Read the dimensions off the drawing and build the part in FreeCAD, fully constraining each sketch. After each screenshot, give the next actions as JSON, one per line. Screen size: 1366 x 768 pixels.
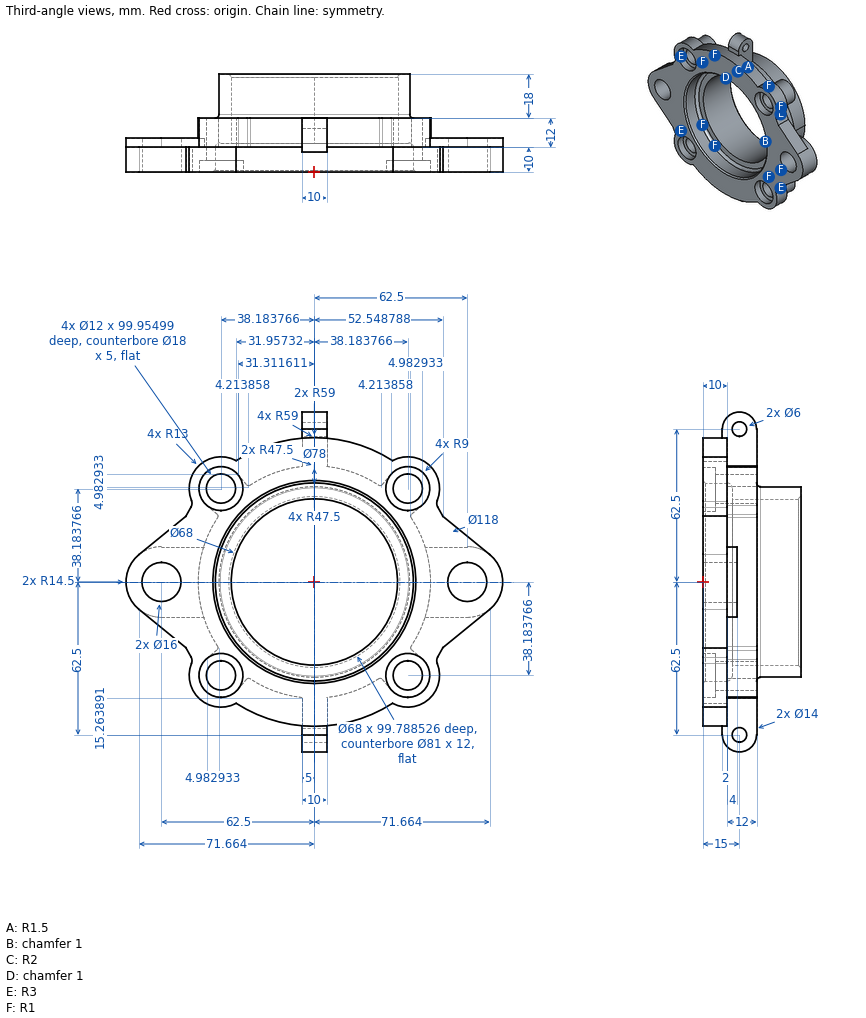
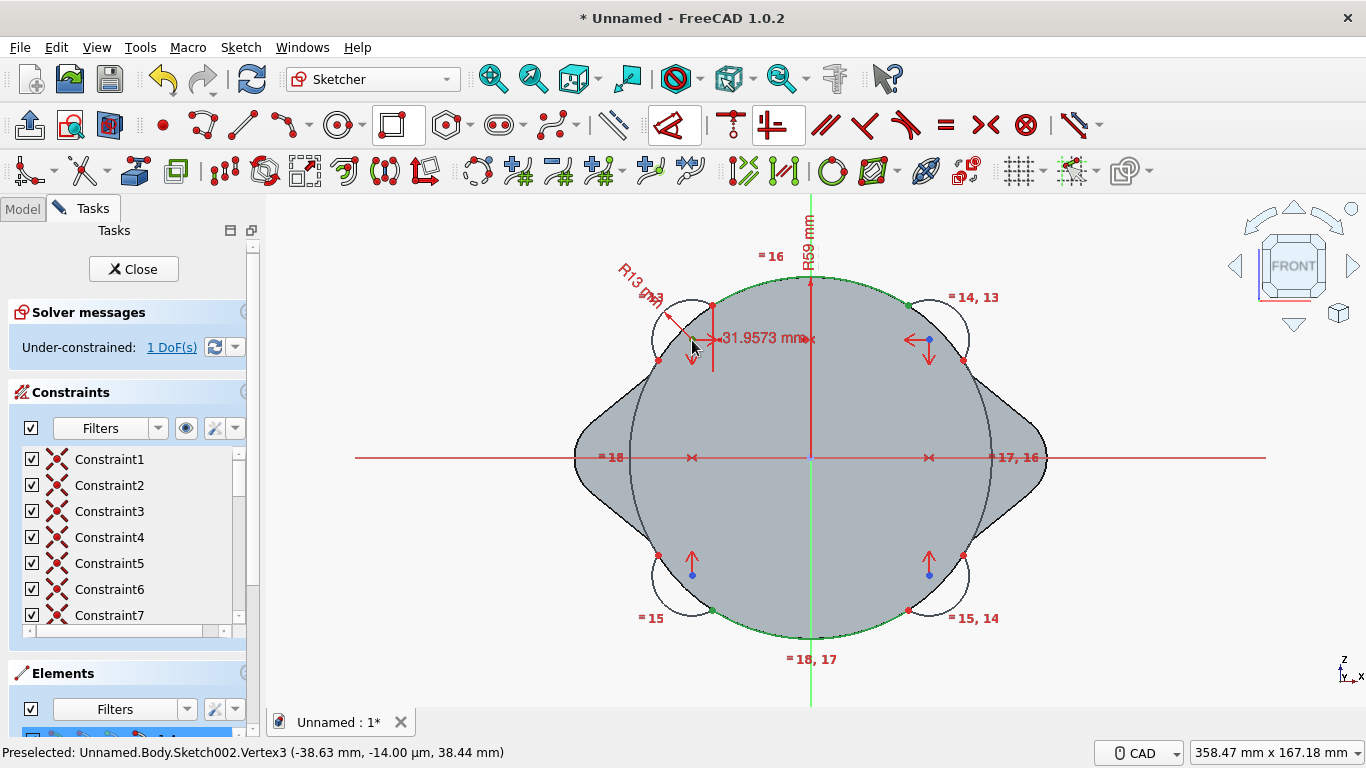
{"action": "key", "text": "l"}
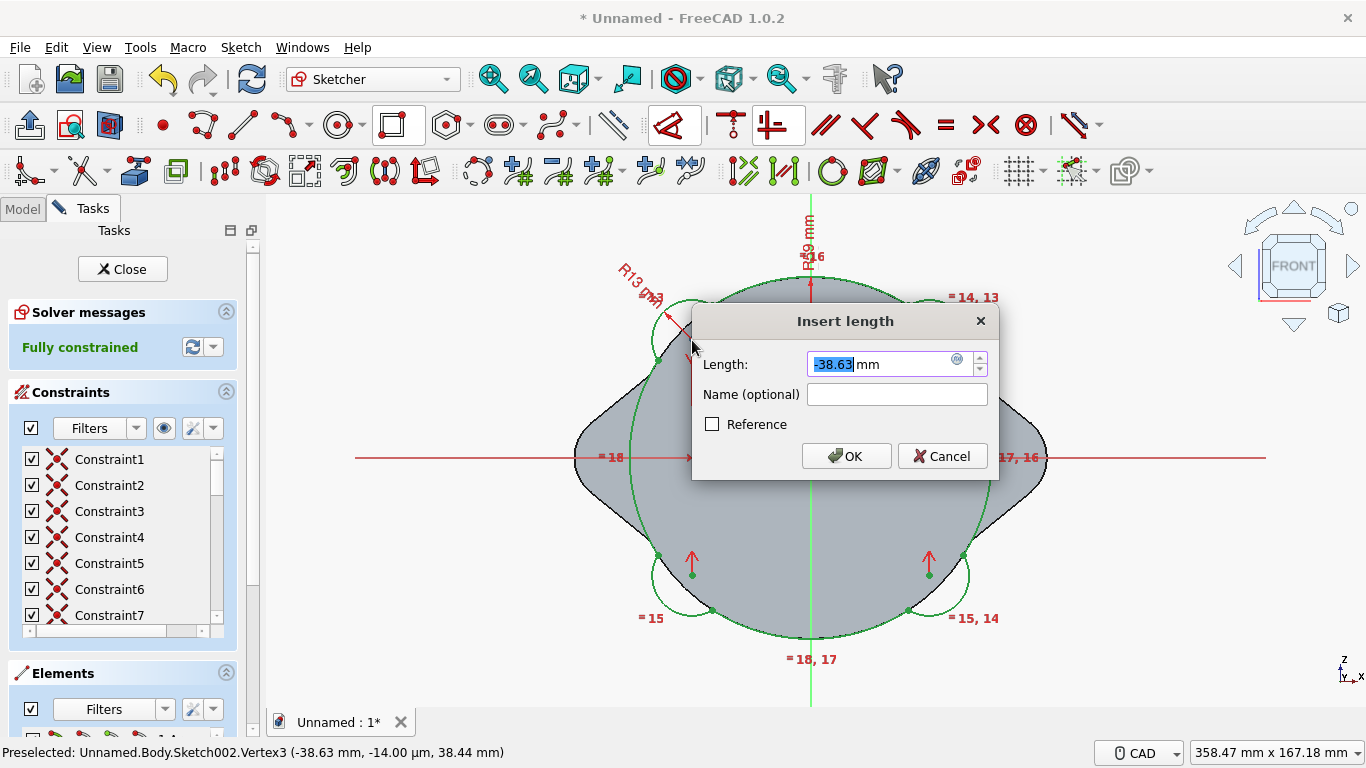
{"action": "type", "text": "-38.183766"}
{"action": "key", "text": "Return"}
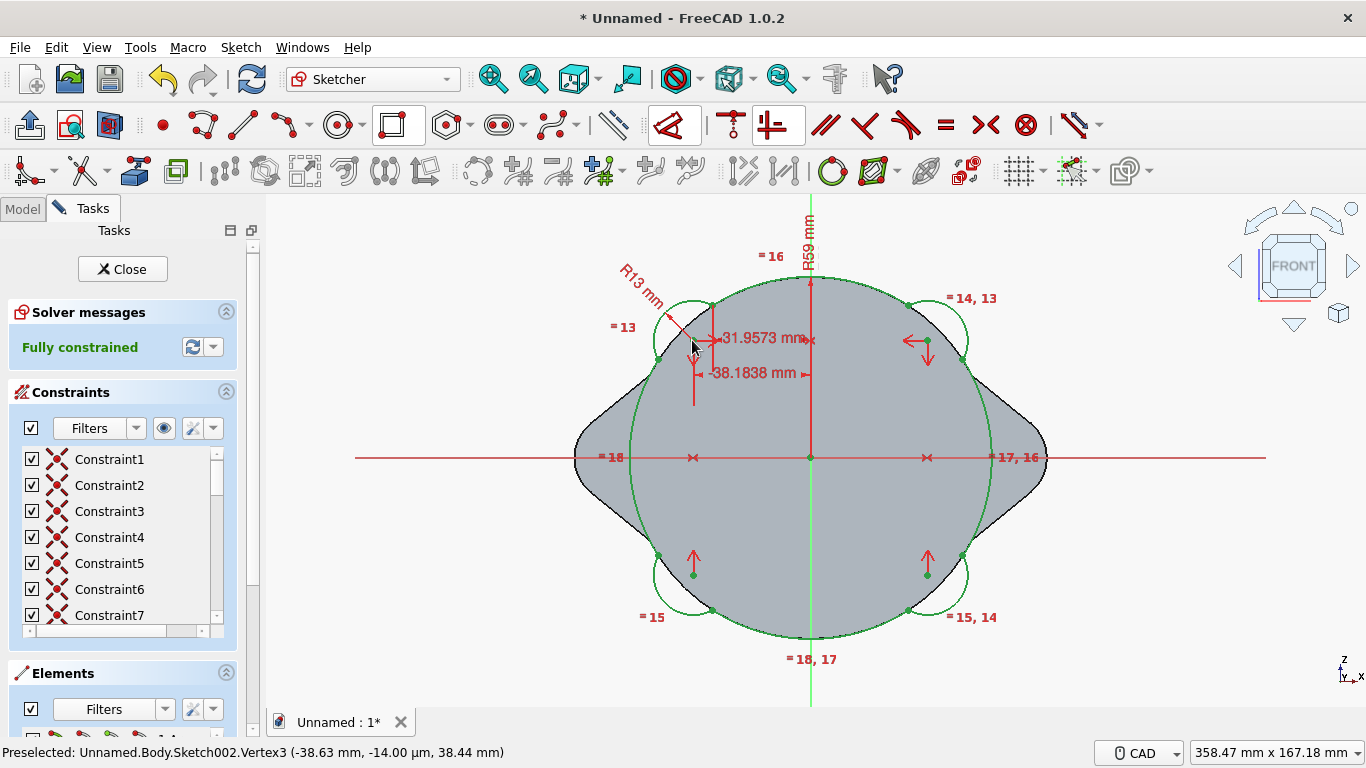
{"action": "left_click", "coordinate": [123, 269]}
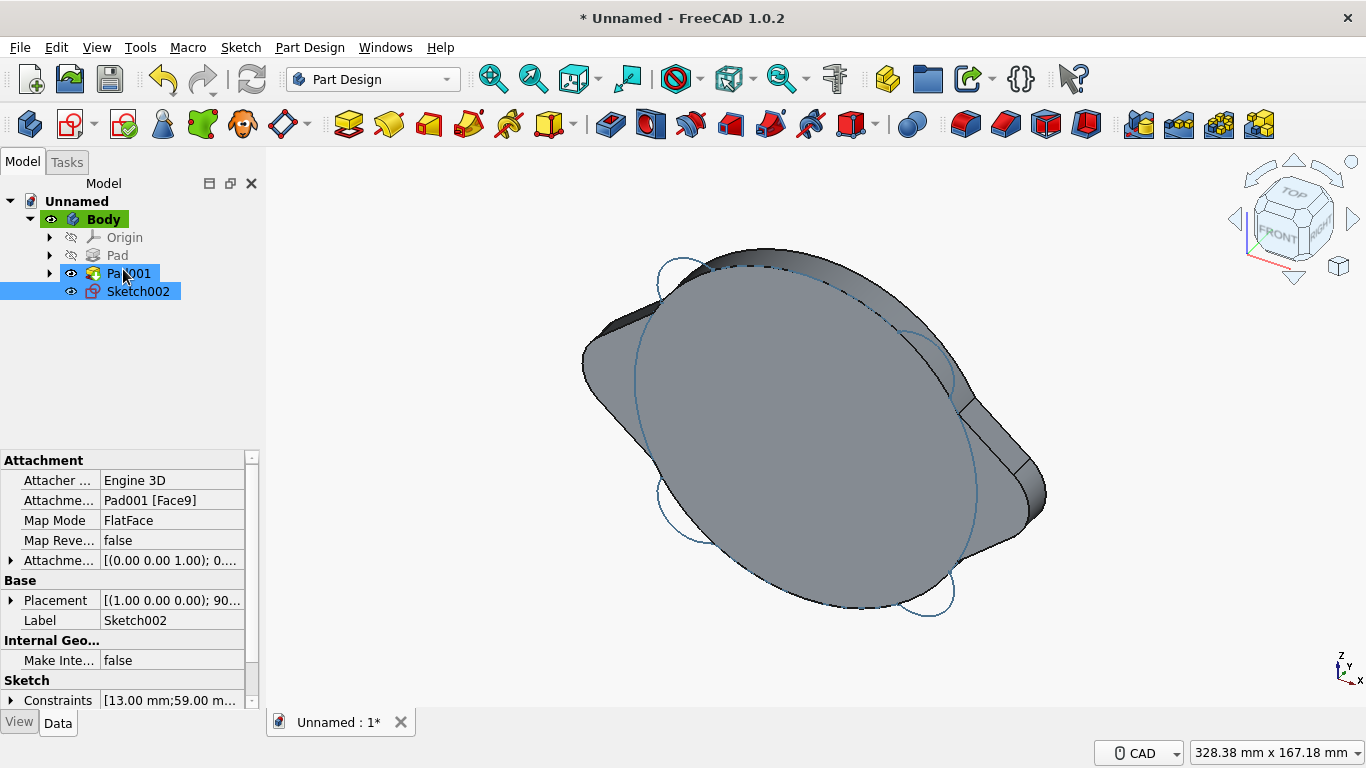
{"action": "left_click", "coordinate": [350, 124]}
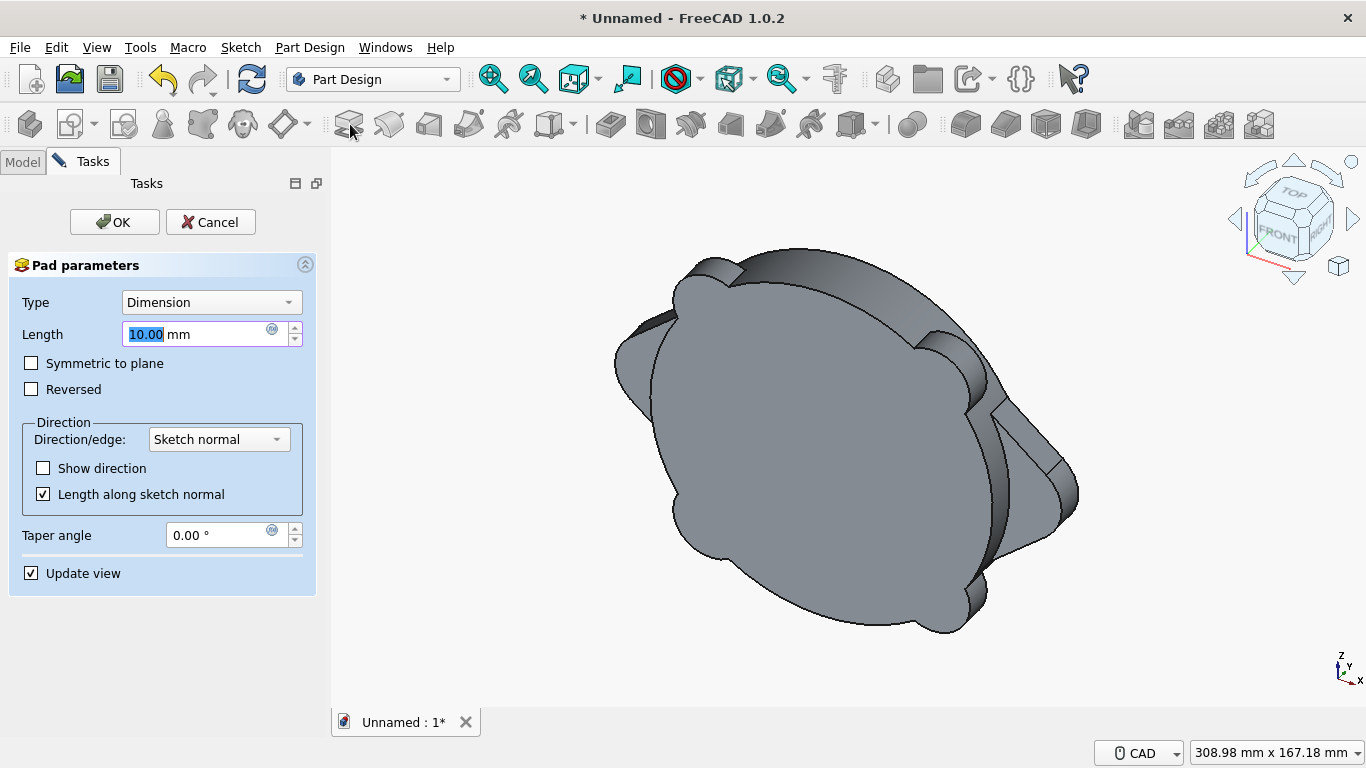
{"action": "type", "text": "10"}
{"action": "key", "text": "Tab"}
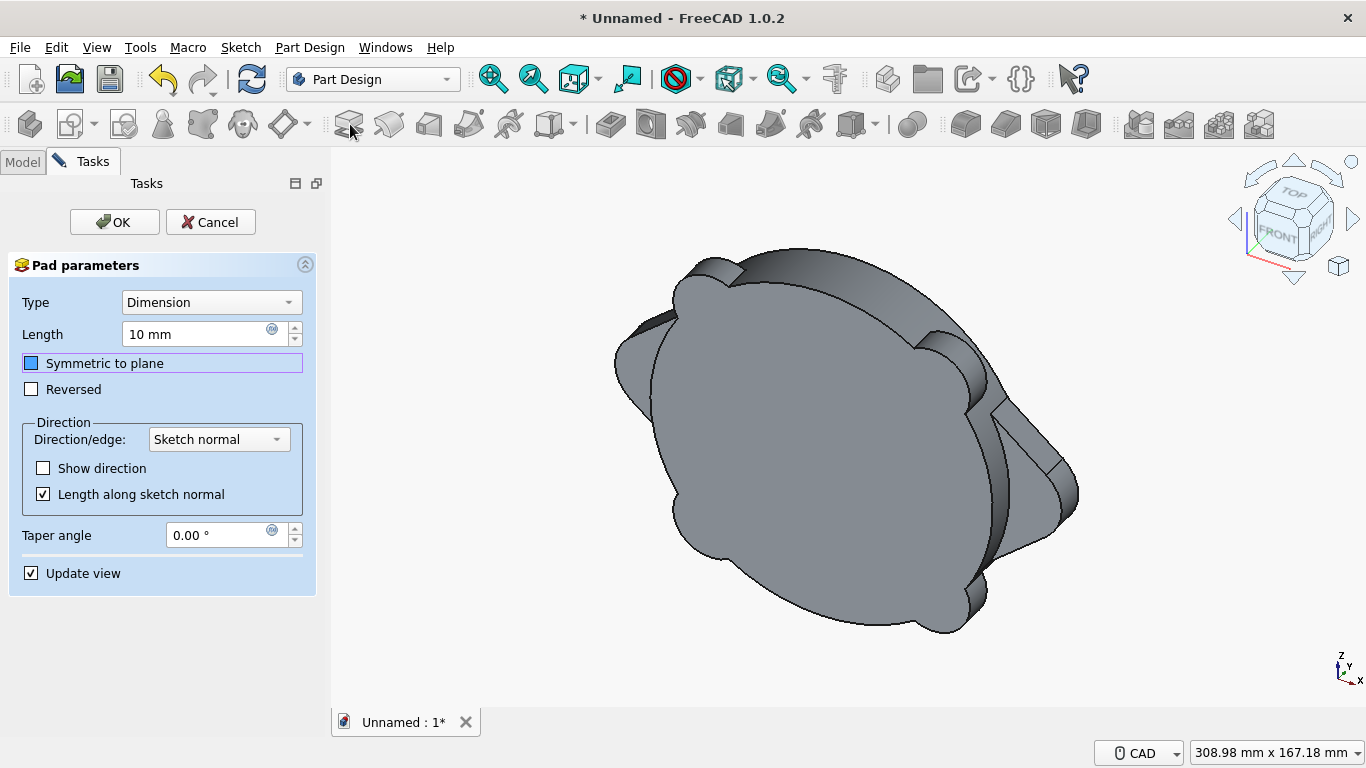
{"action": "left_click", "coordinate": [30, 389]}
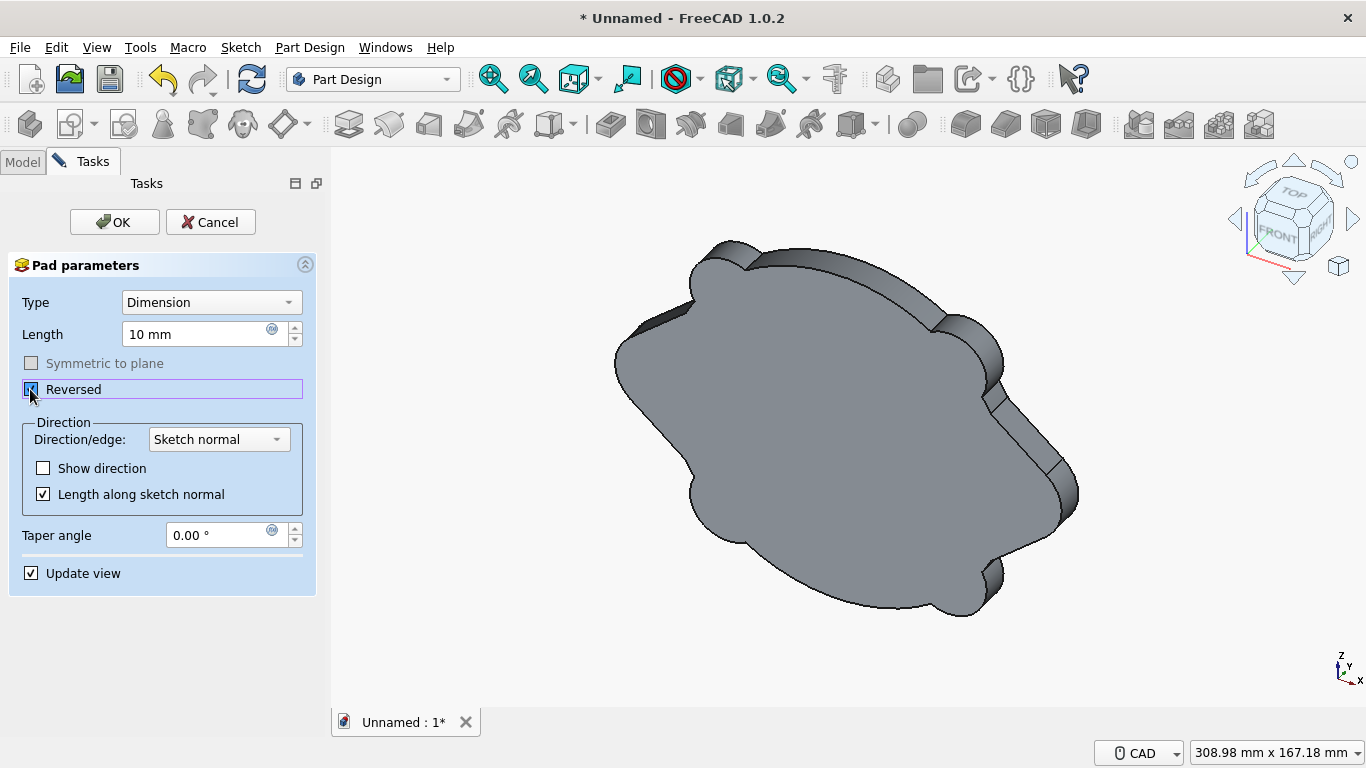
{"action": "left_click", "coordinate": [115, 222]}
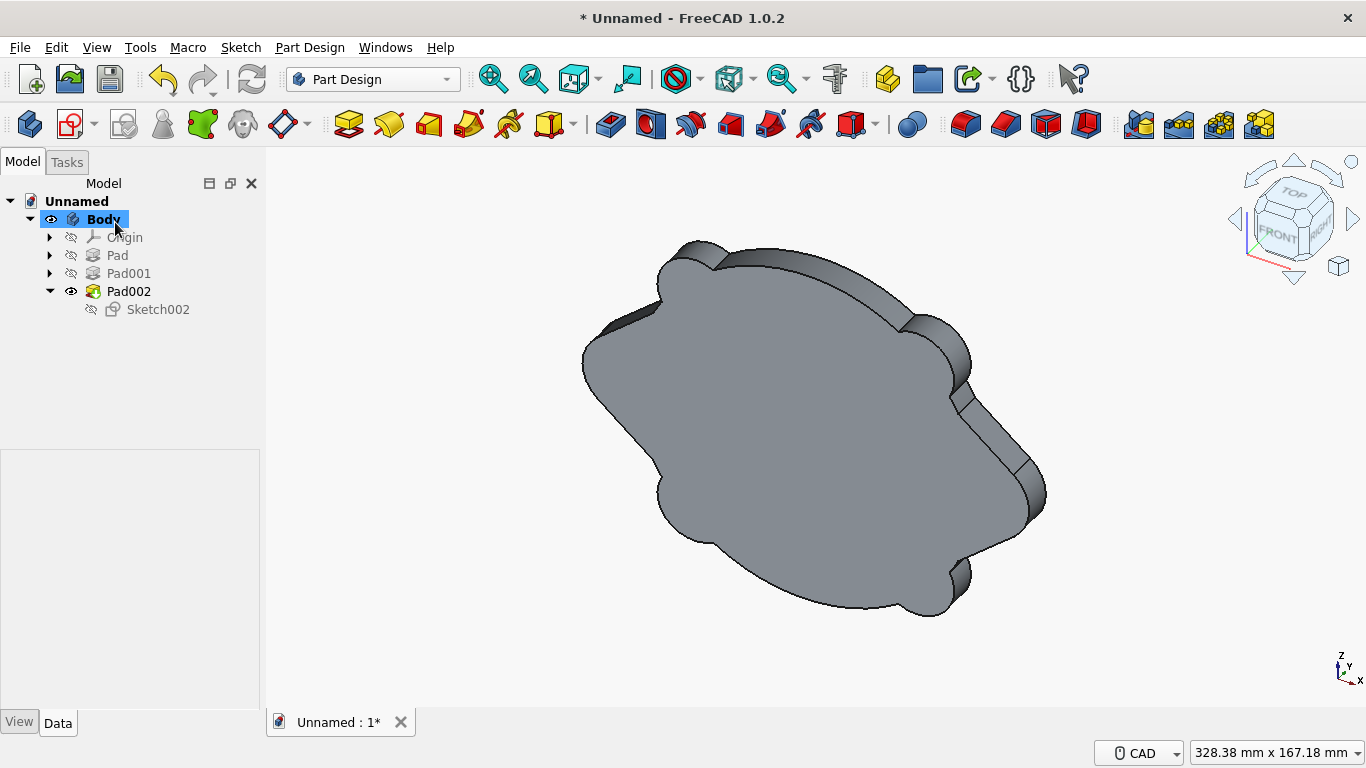
{"action": "key", "text": "4"}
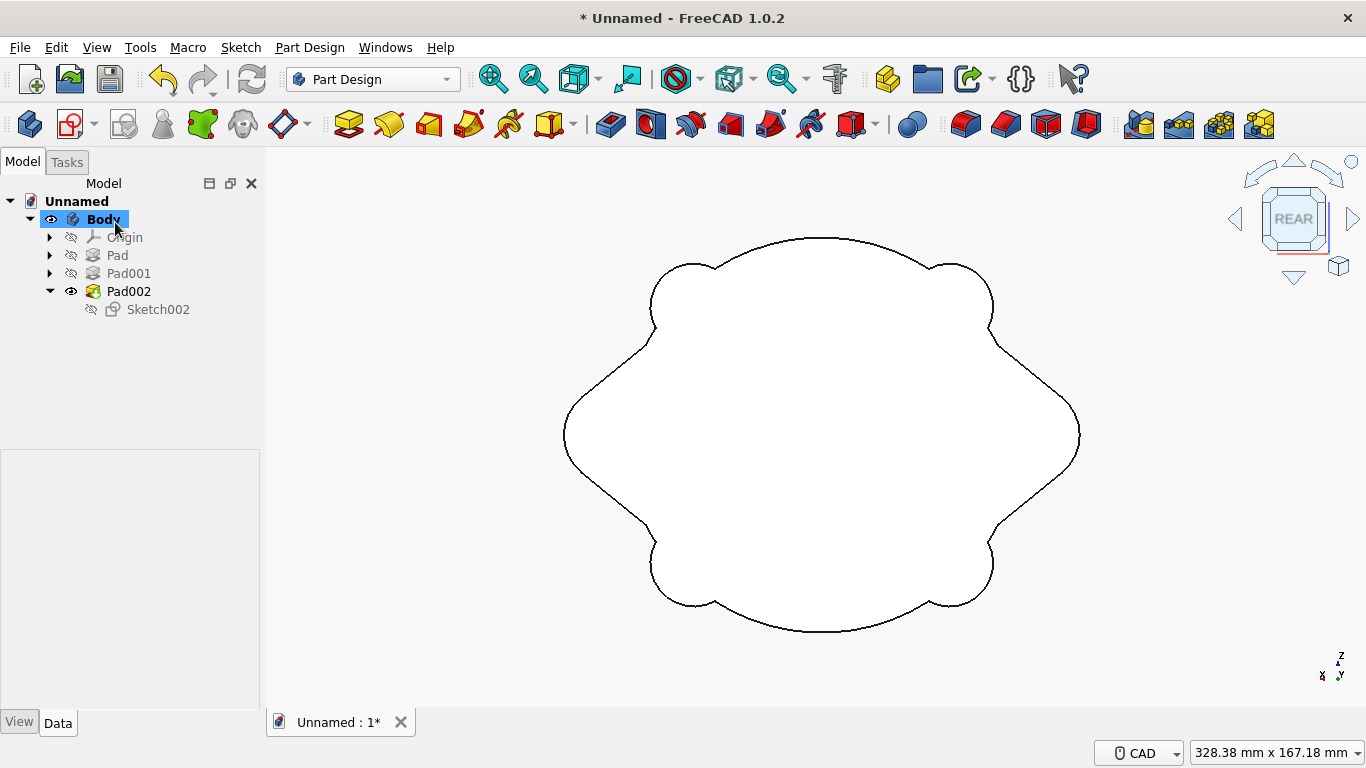
{"action": "left_click", "coordinate": [822, 434]}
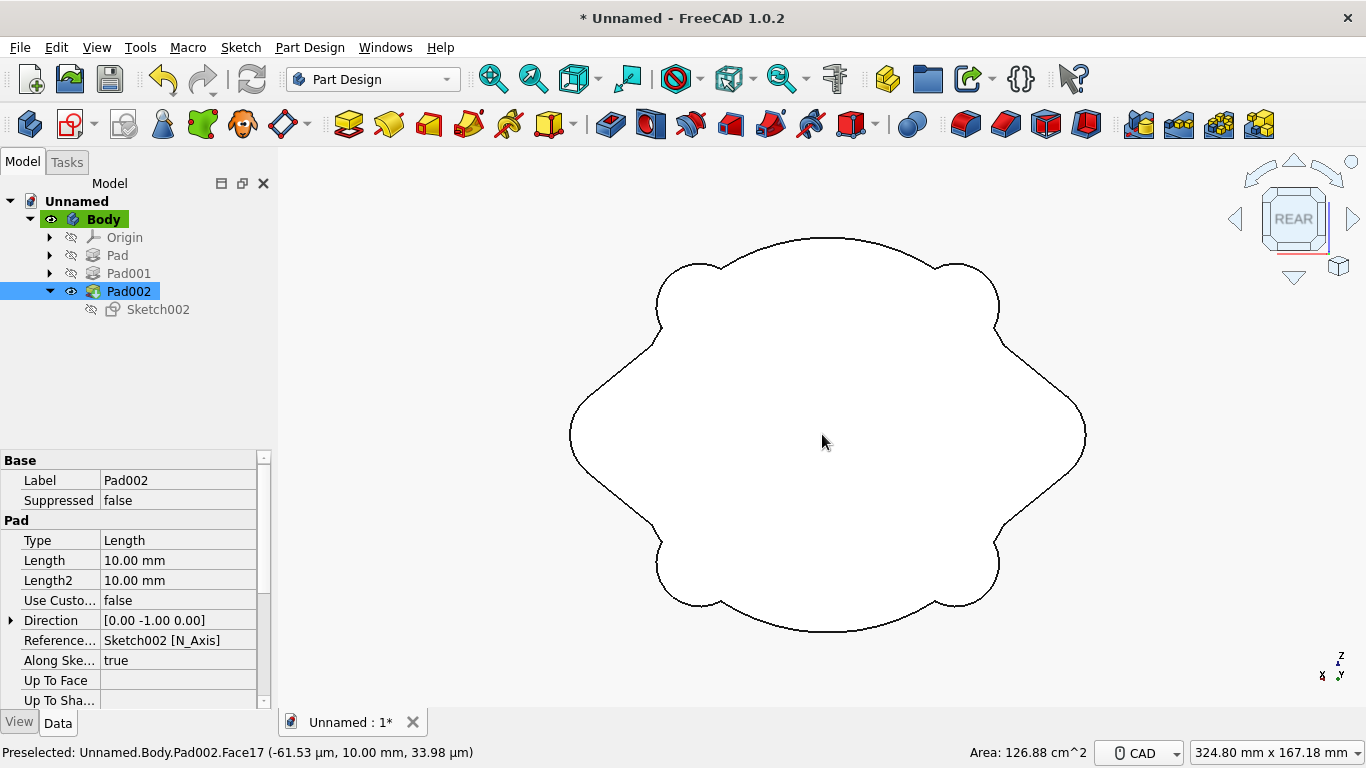
{"action": "left_click", "coordinate": [70, 124]}